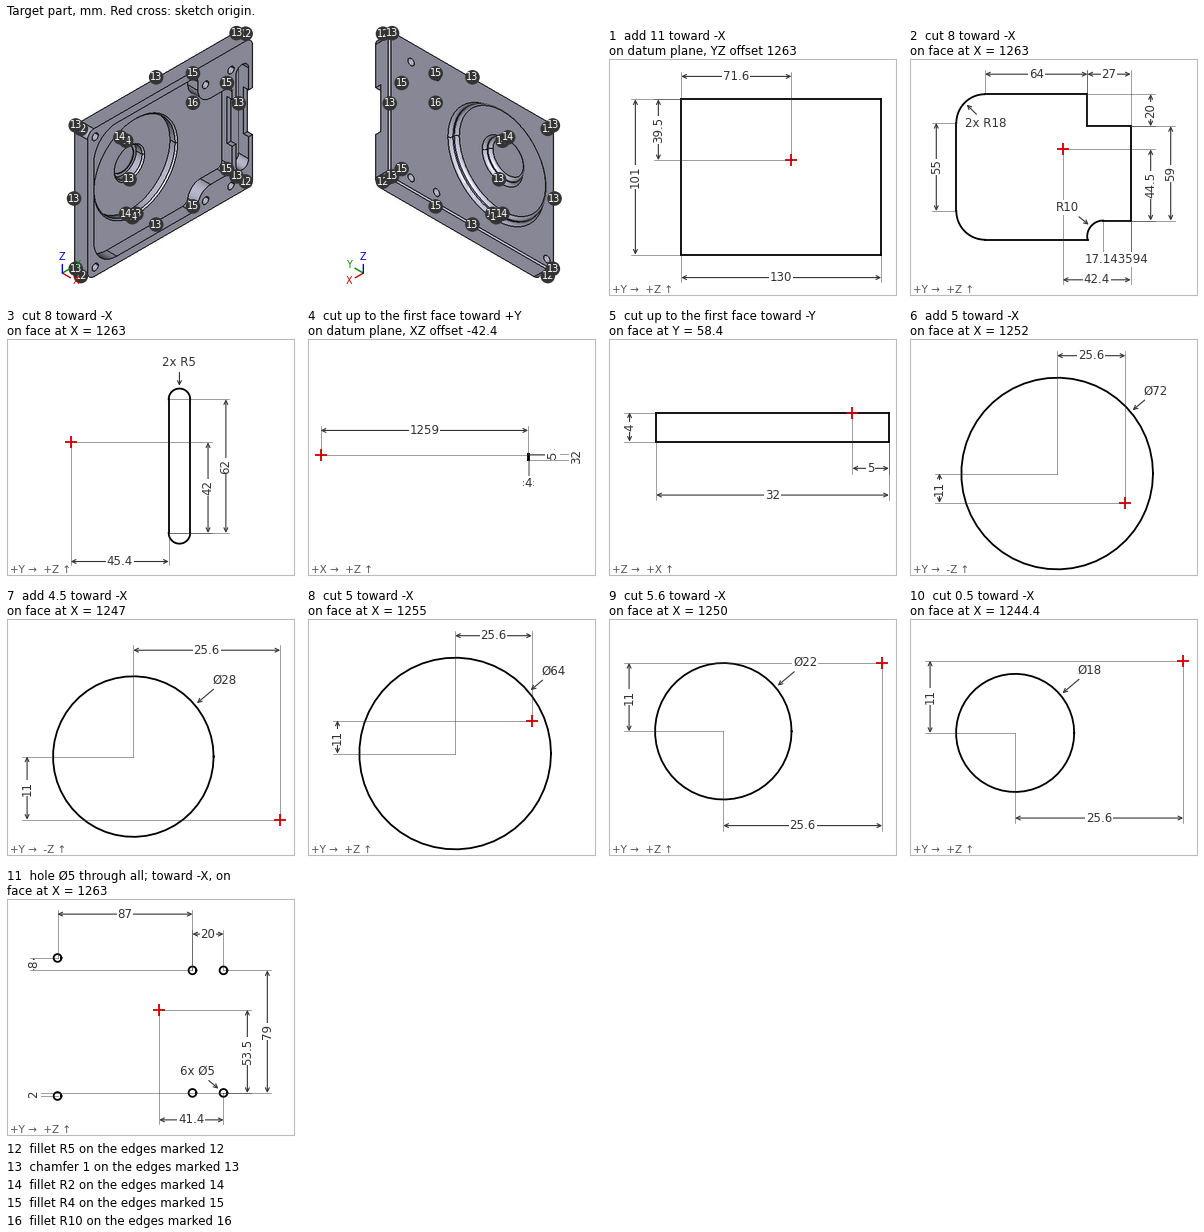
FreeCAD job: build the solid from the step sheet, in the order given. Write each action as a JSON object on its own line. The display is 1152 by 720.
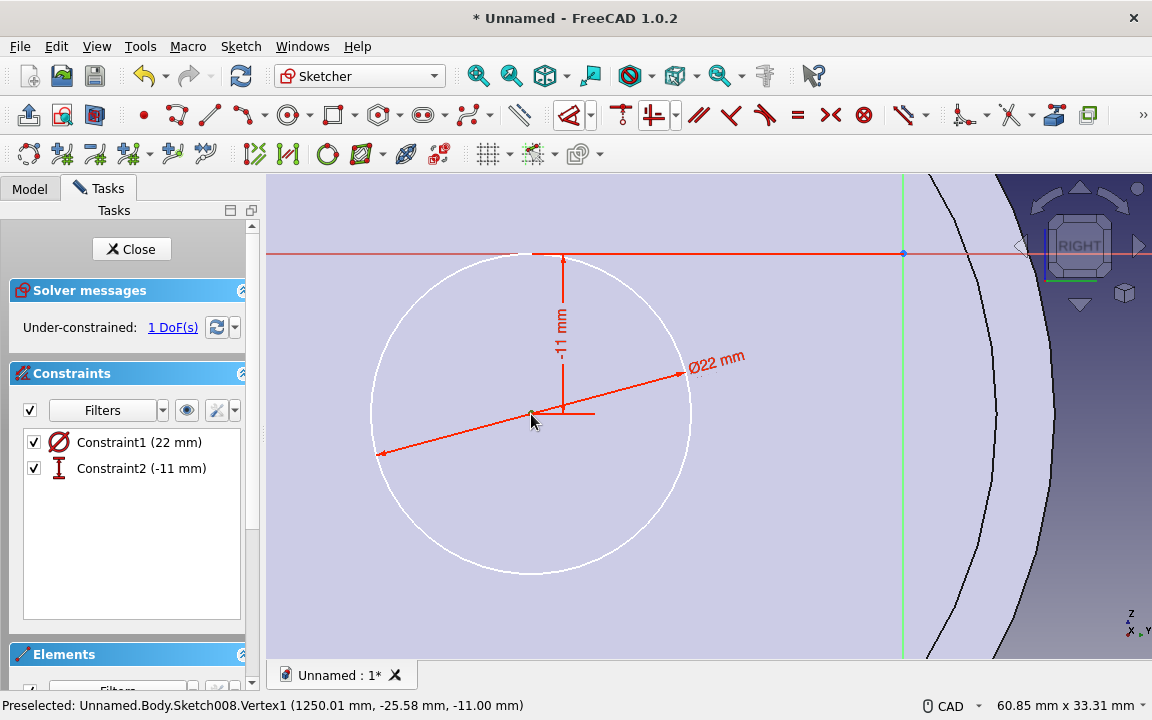
{"action": "key", "text": "l"}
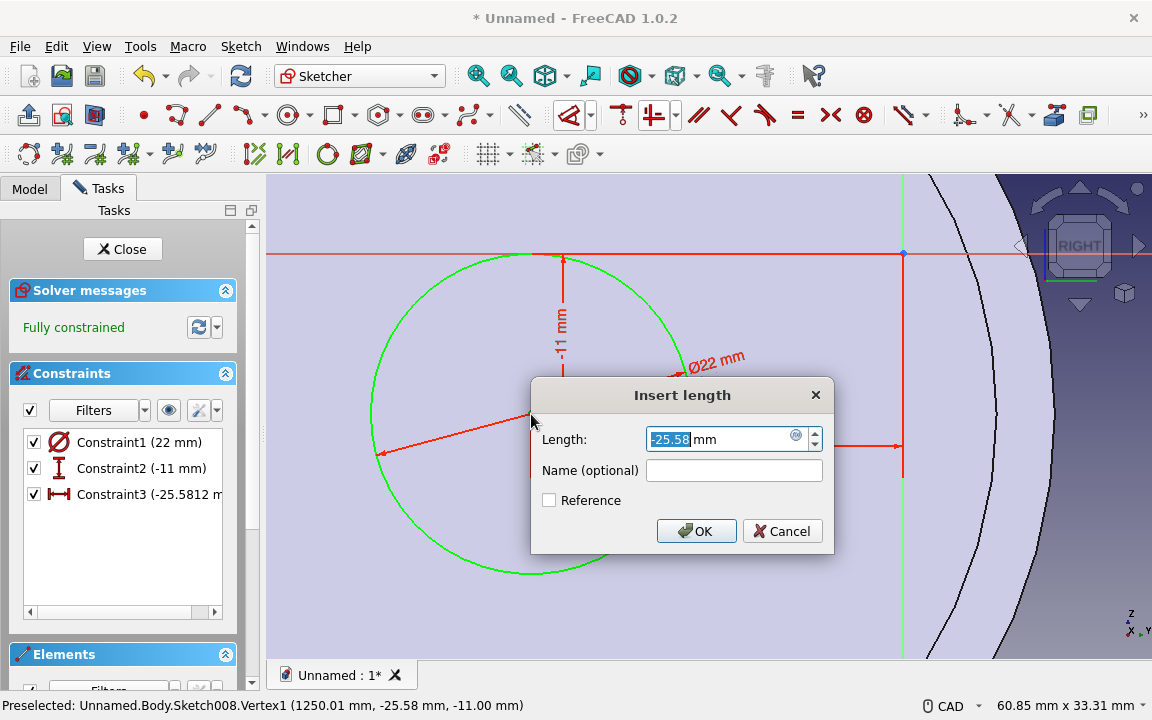
{"action": "type", "text": "-25.6"}
{"action": "key", "text": "Return"}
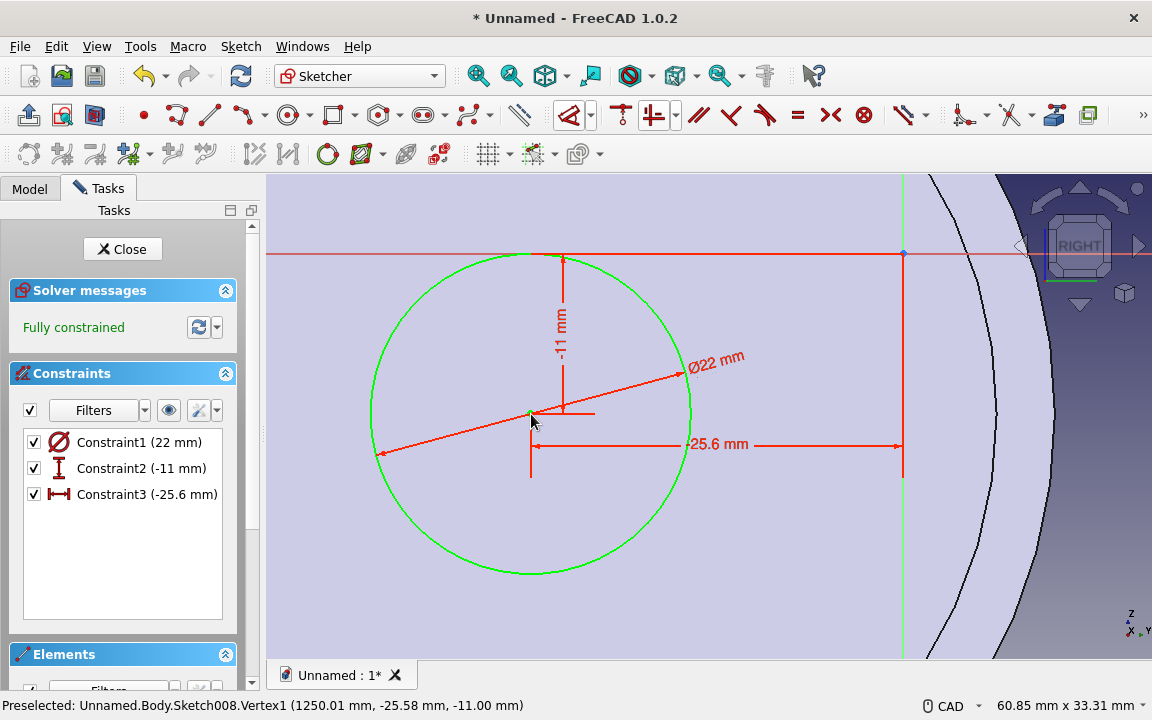
{"action": "left_click", "coordinate": [123, 249]}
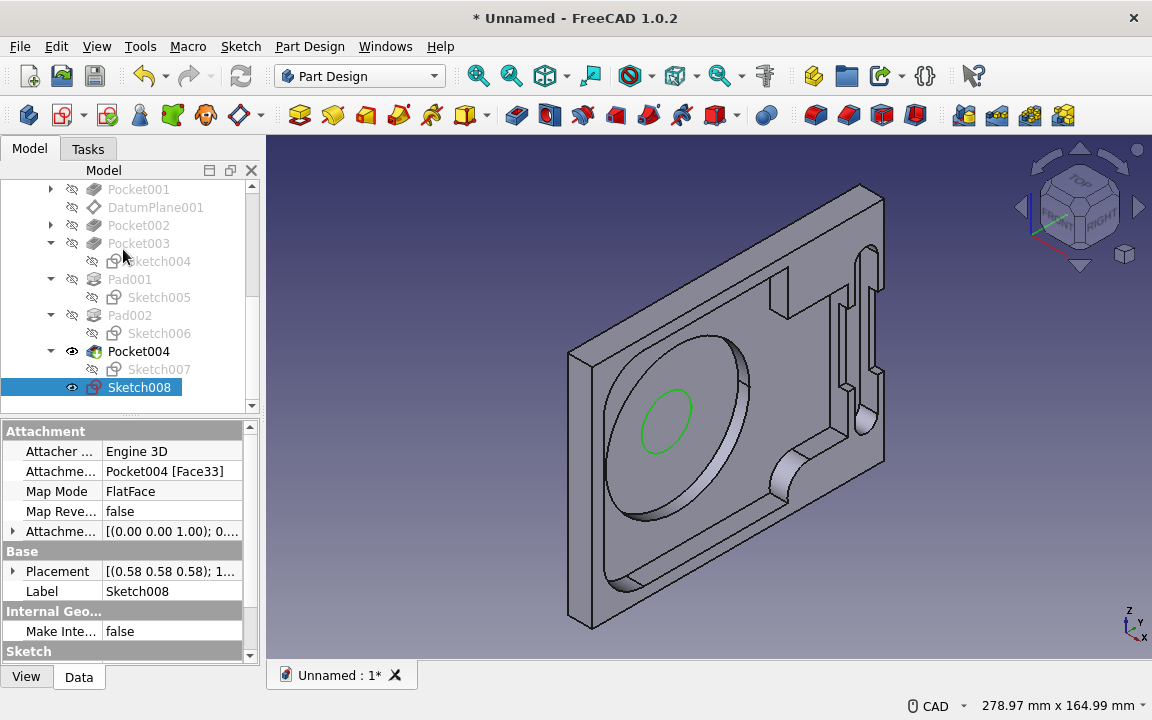
{"action": "left_click", "coordinate": [517, 116]}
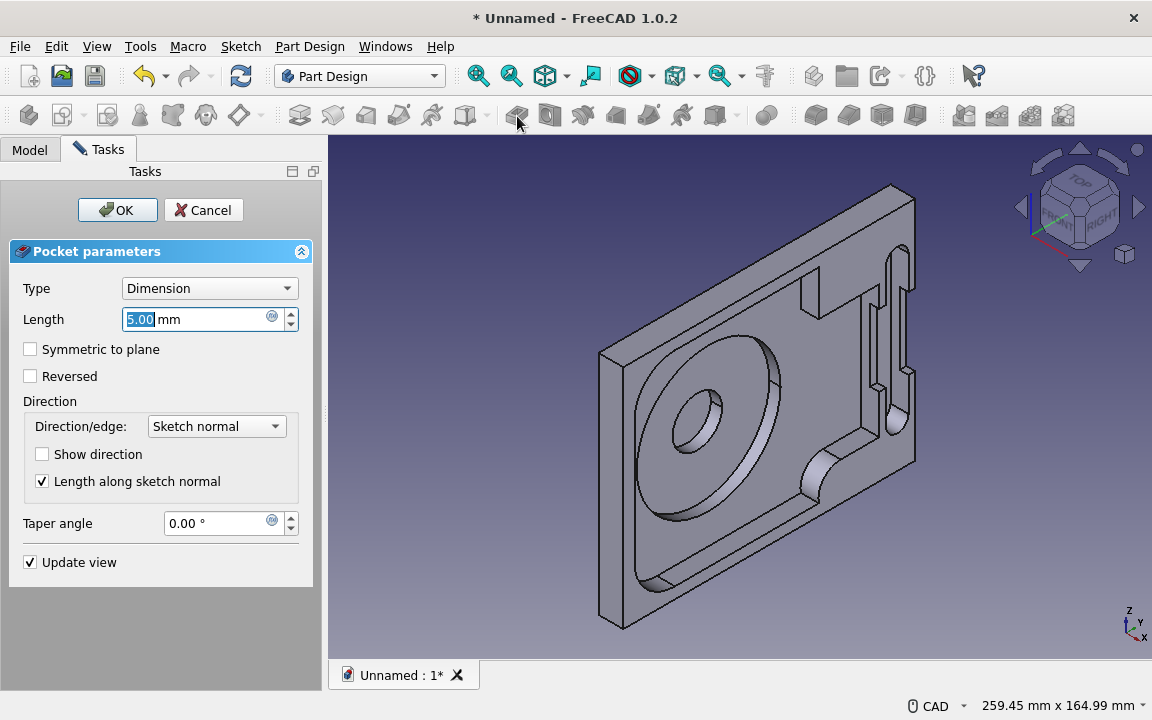
{"action": "type", "text": "5.6"}
{"action": "key", "text": "Tab"}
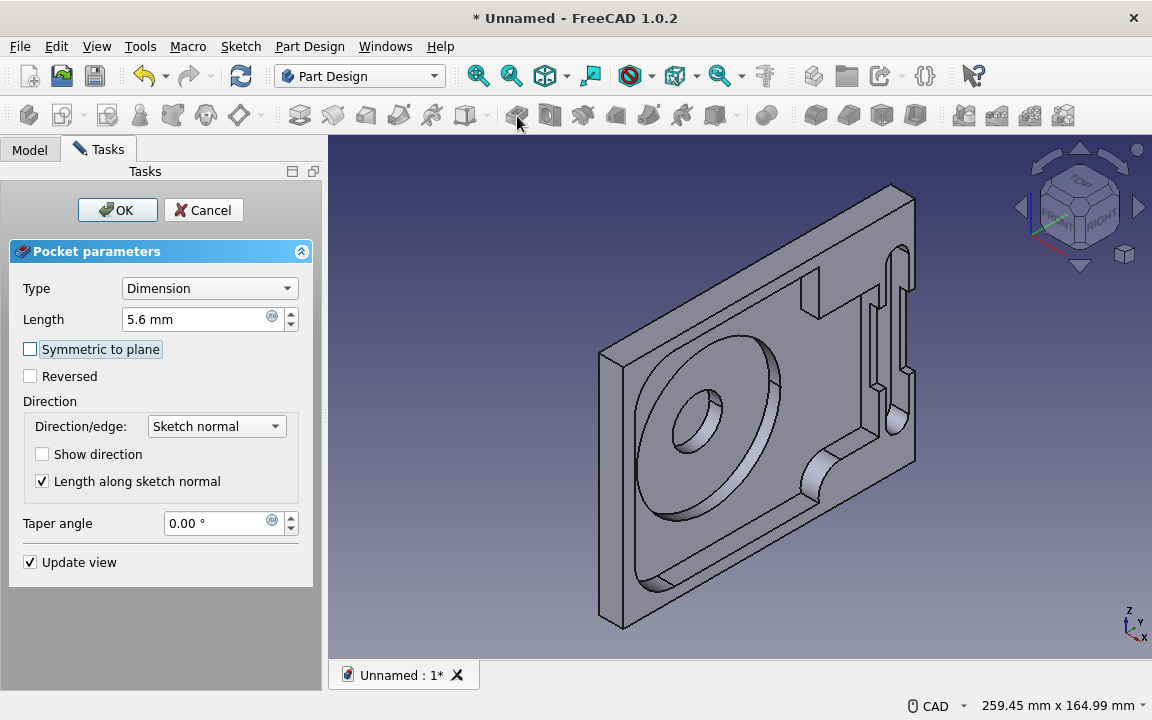
{"action": "left_click", "coordinate": [118, 210]}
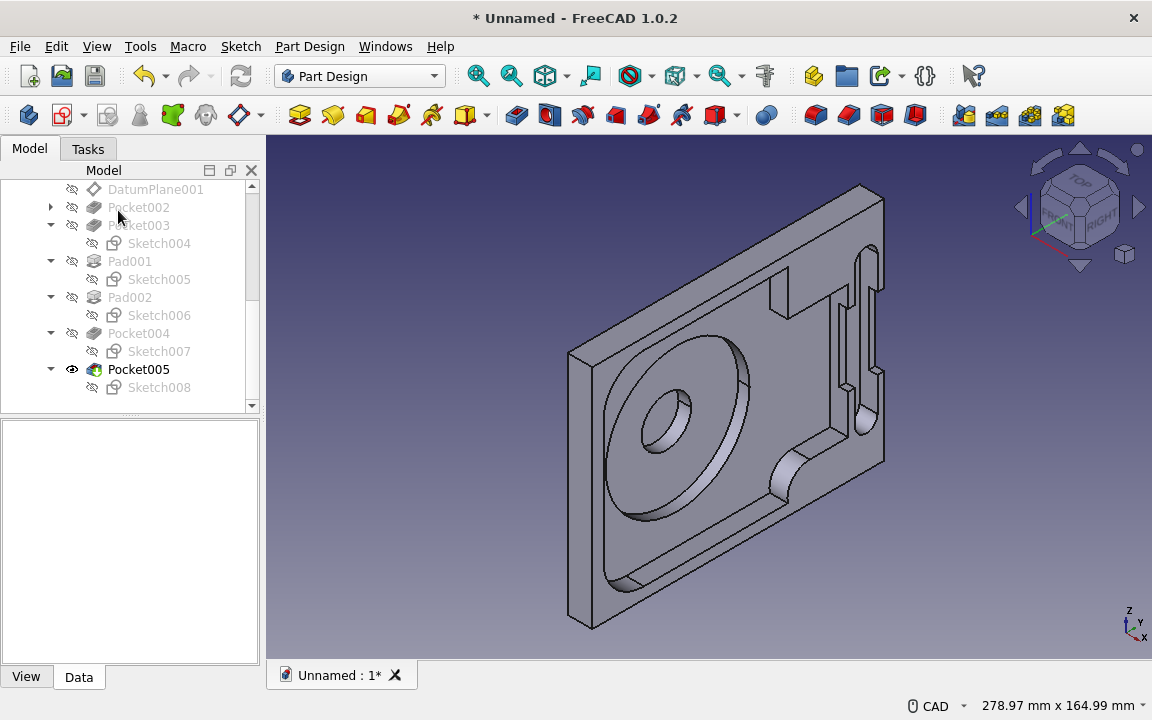
{"action": "left_click", "coordinate": [654, 422]}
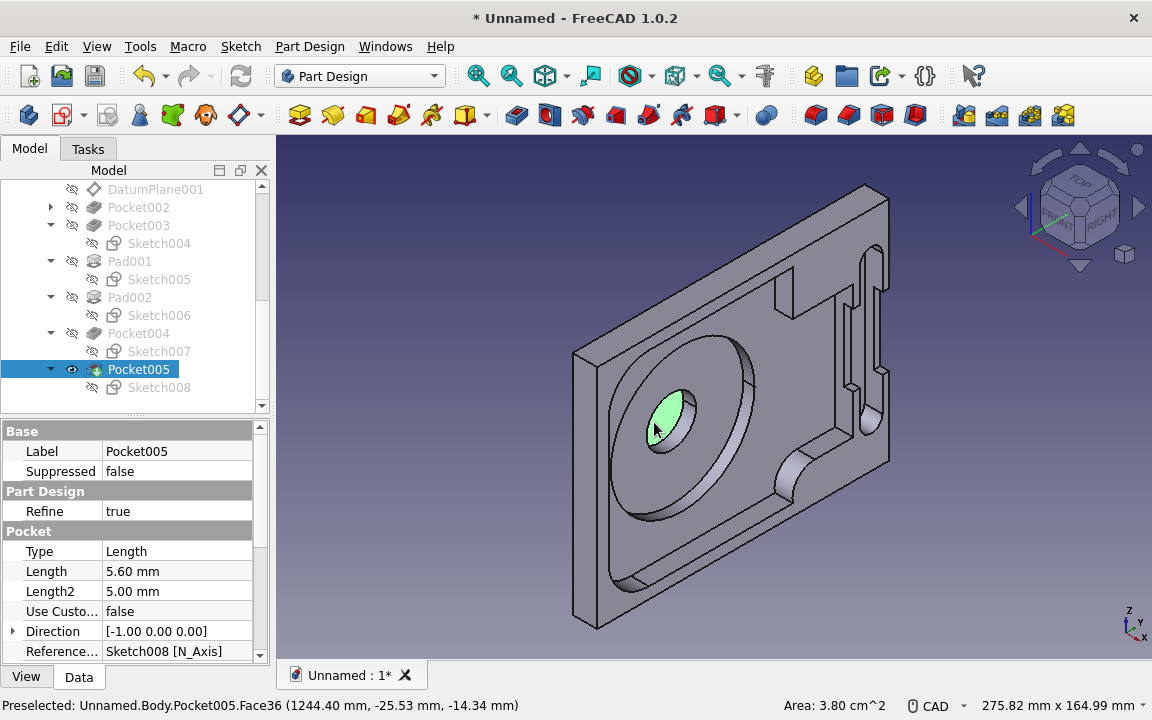
{"action": "left_click", "coordinate": [62, 116]}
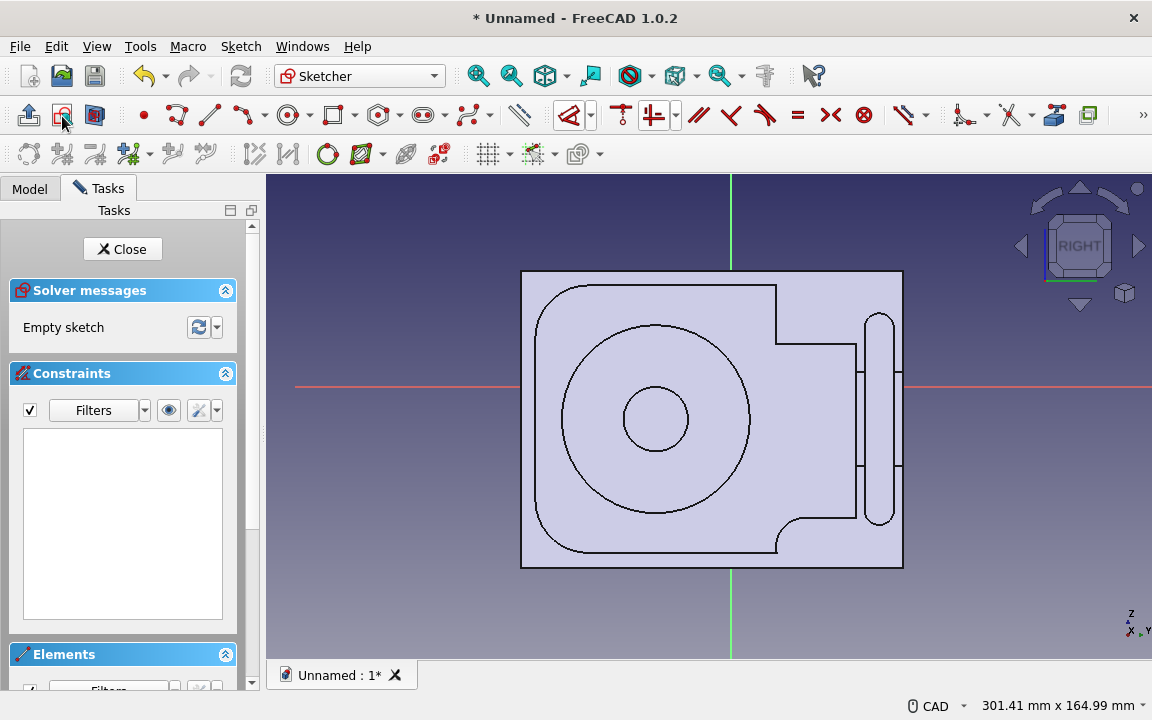
{"action": "scroll", "coordinate": [690, 416], "scroll_direction": "up", "scroll_amount": 8}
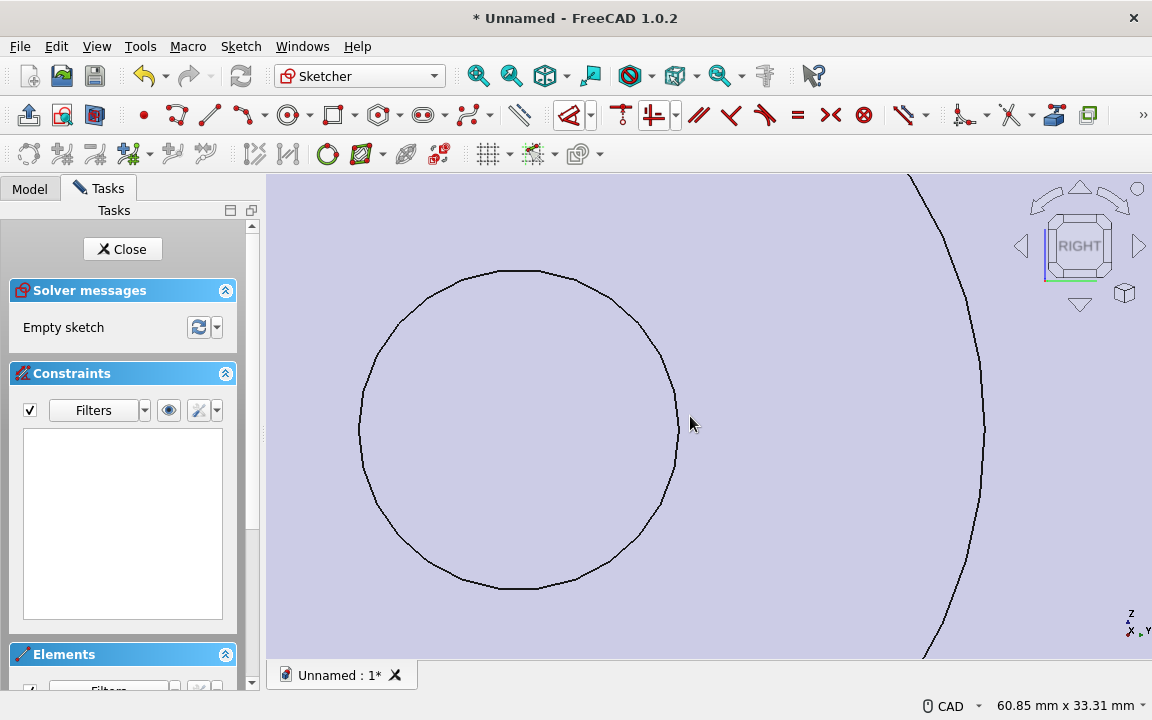
{"action": "left_click", "coordinate": [288, 116]}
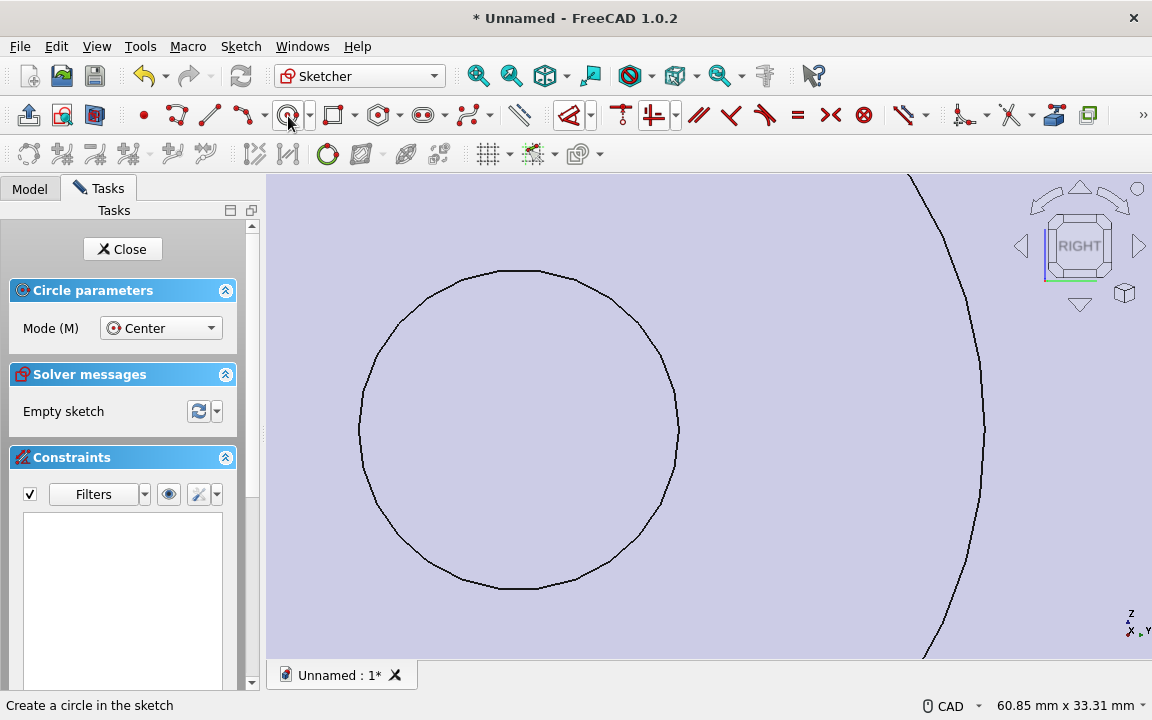
{"action": "left_click", "coordinate": [519, 430]}
{"action": "left_click", "coordinate": [612, 337]}
{"action": "key", "text": "Escape"}